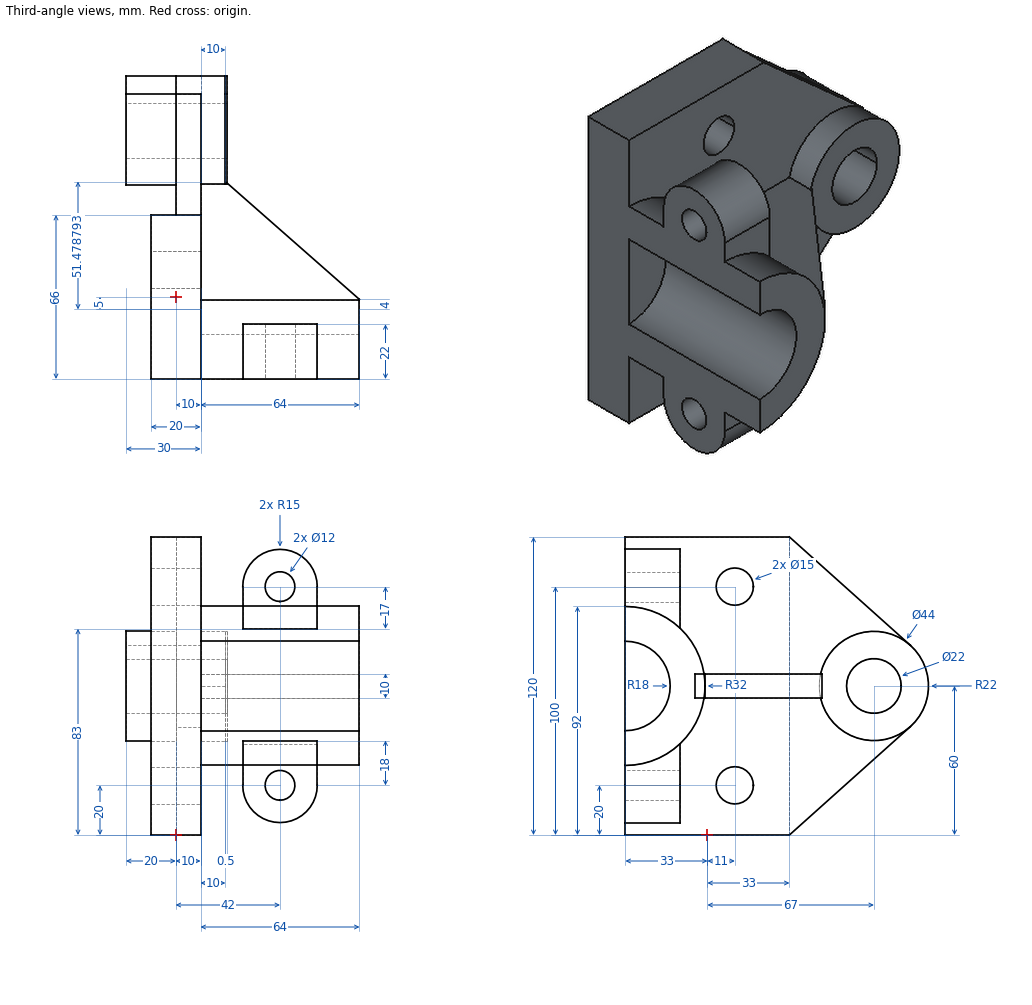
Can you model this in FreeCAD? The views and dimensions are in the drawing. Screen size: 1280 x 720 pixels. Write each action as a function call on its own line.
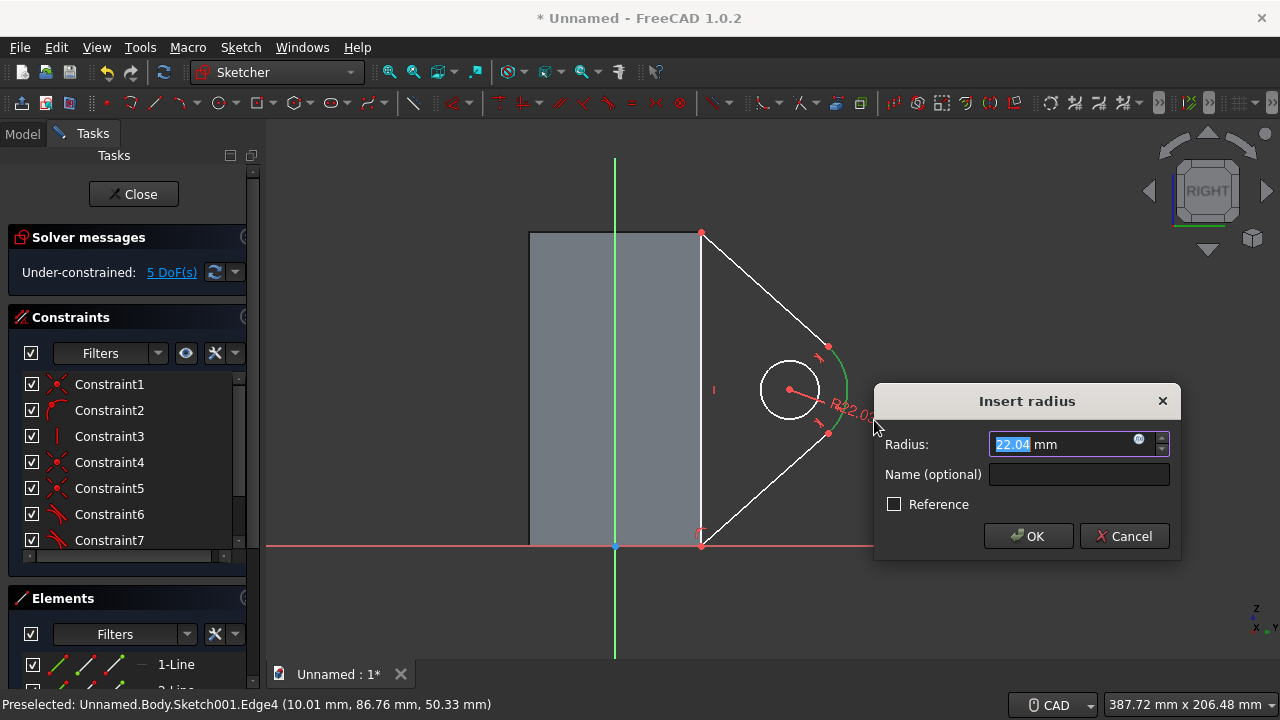
text(22)
key(Return)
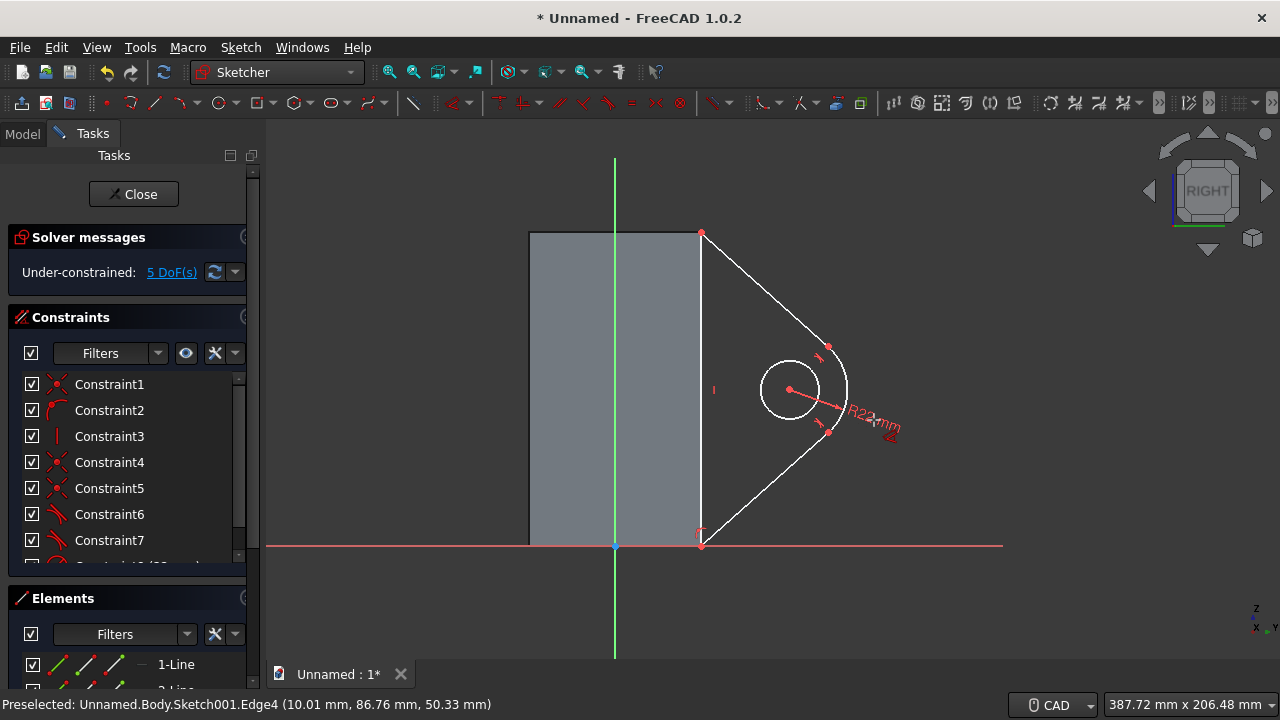
click(810, 369)
click(776, 331)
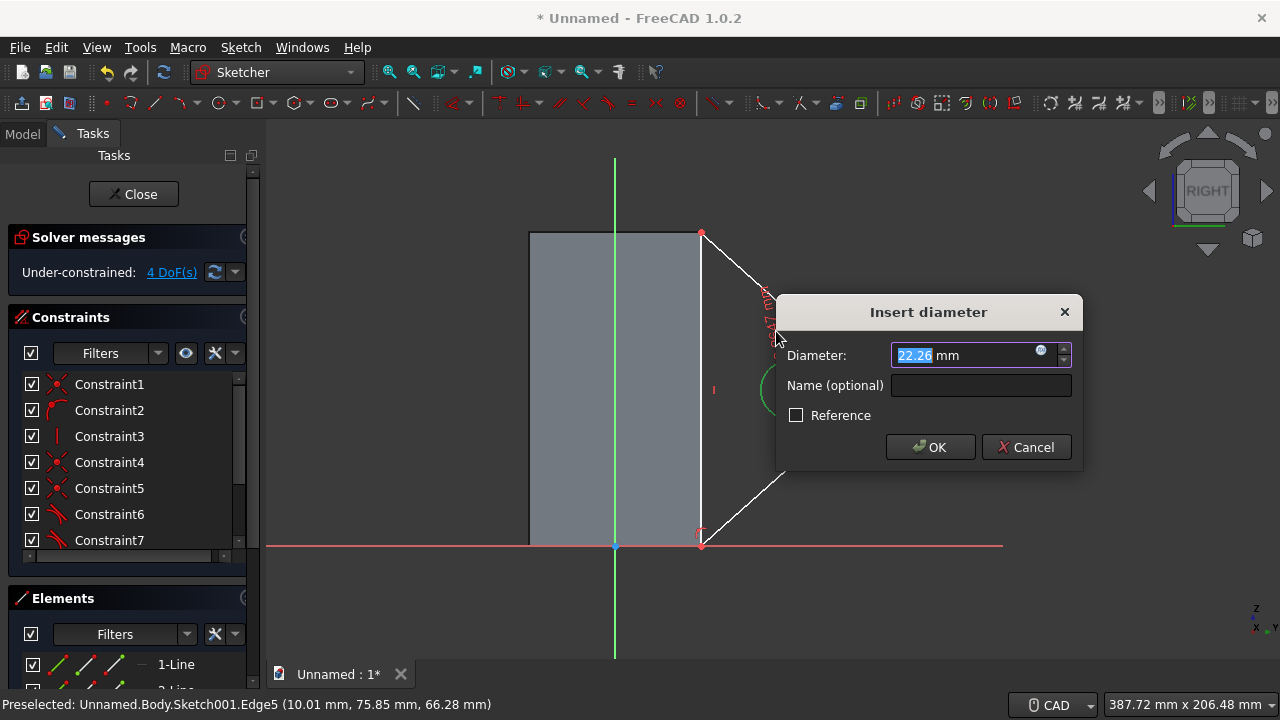
text(22)
key(Return)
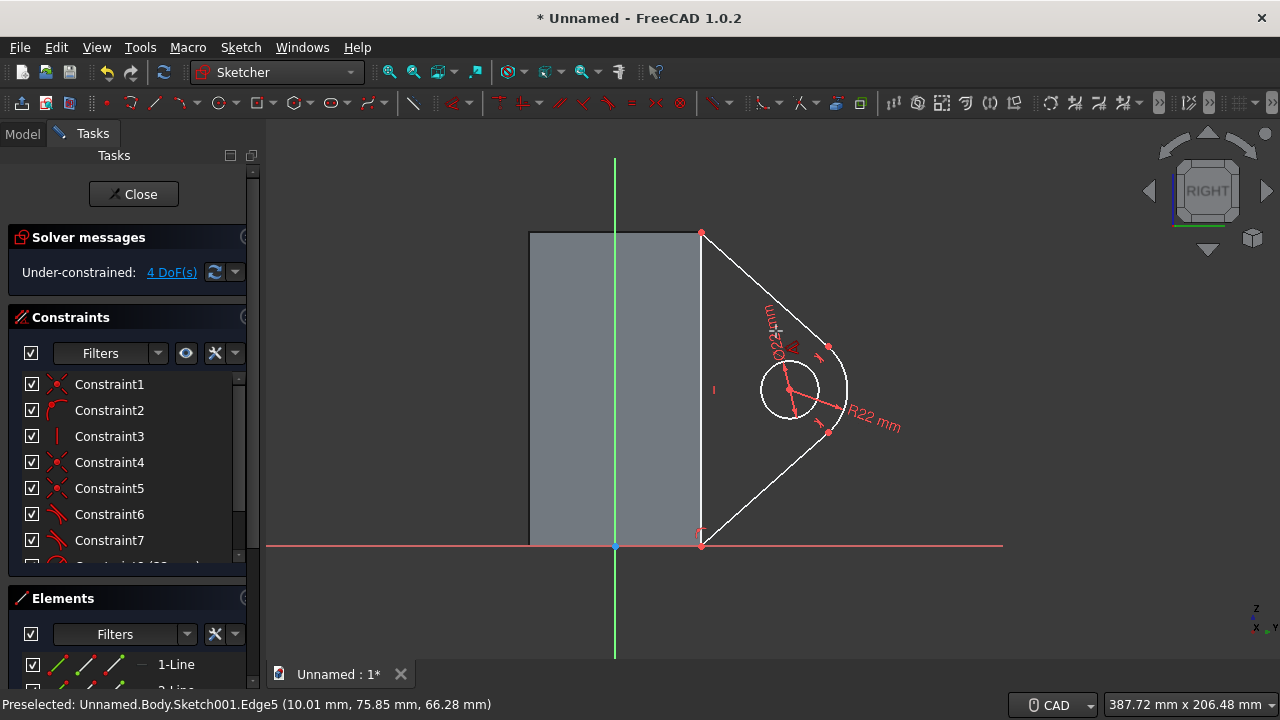
click(790, 390)
click(703, 580)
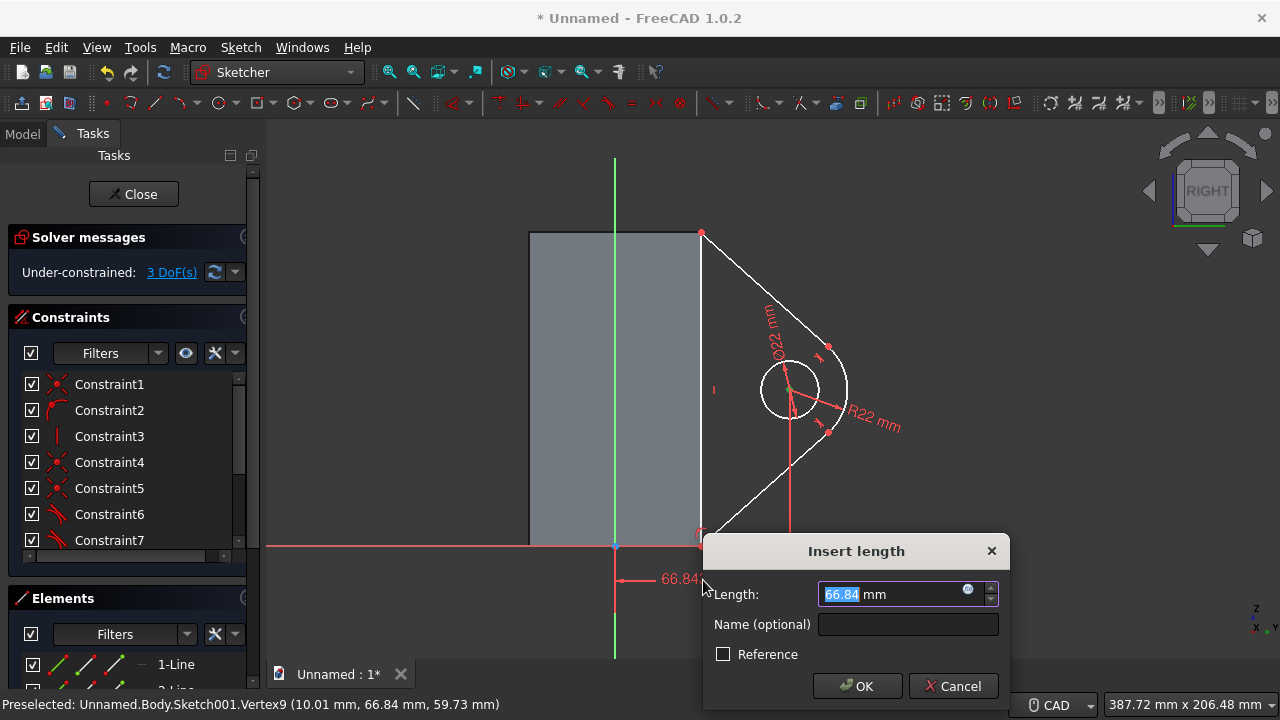
text(67)
key(Return)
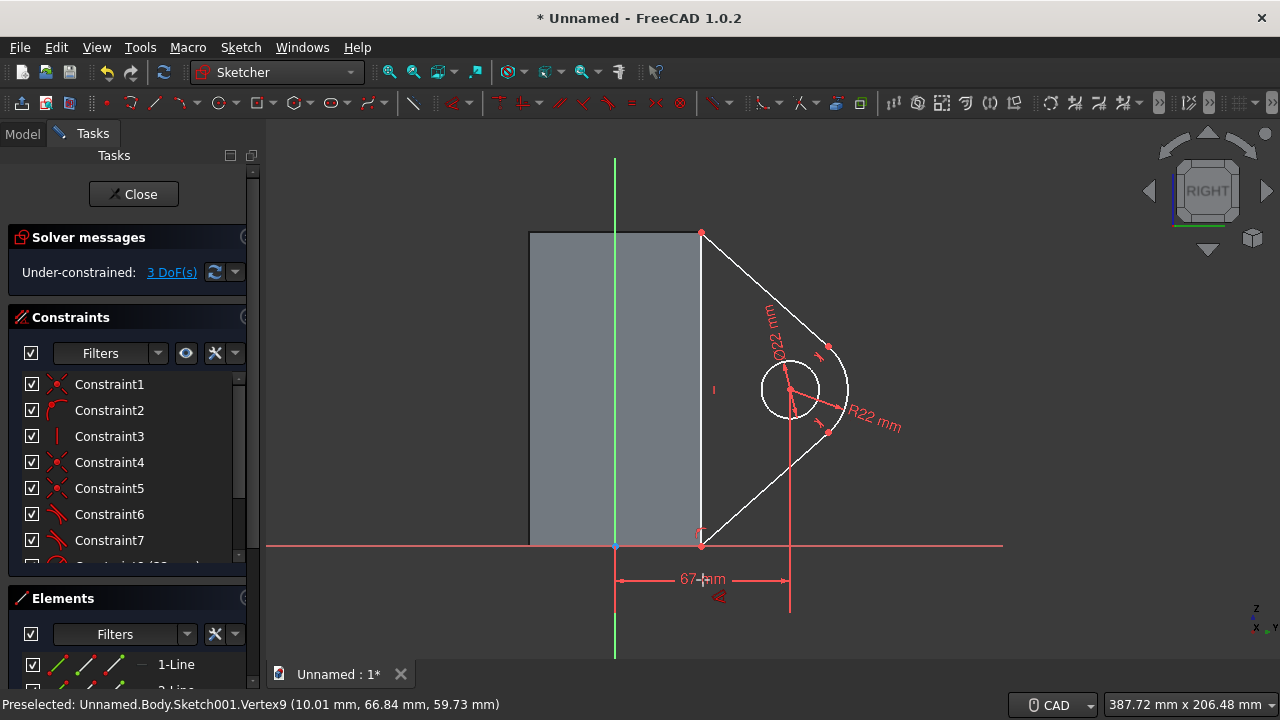
click(790, 390)
click(581, 468)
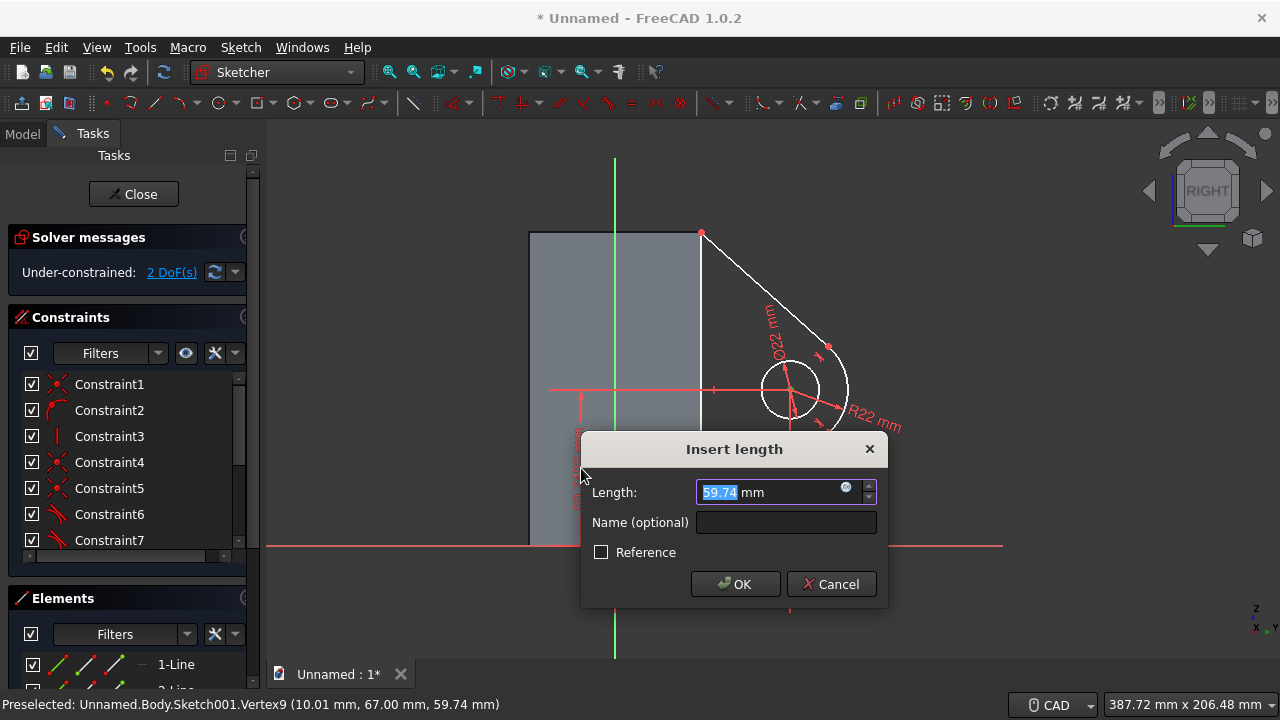
text(60)
key(Return)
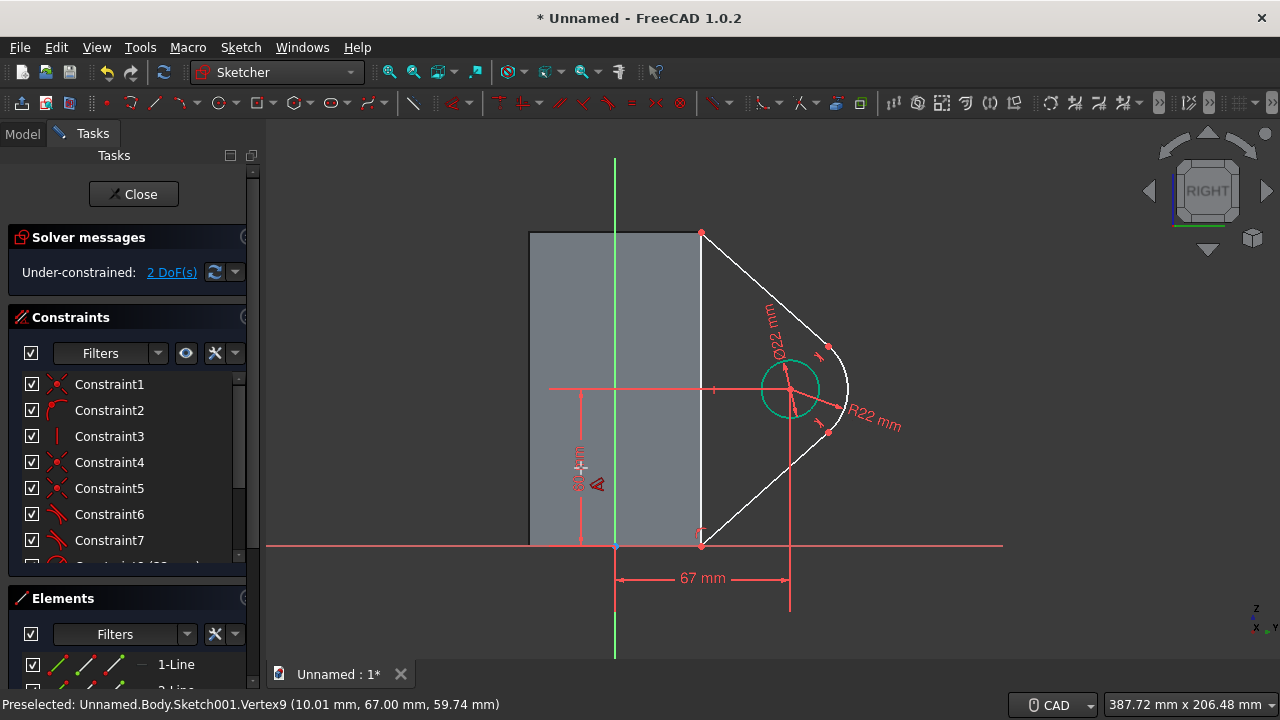
click(701, 327)
click(667, 390)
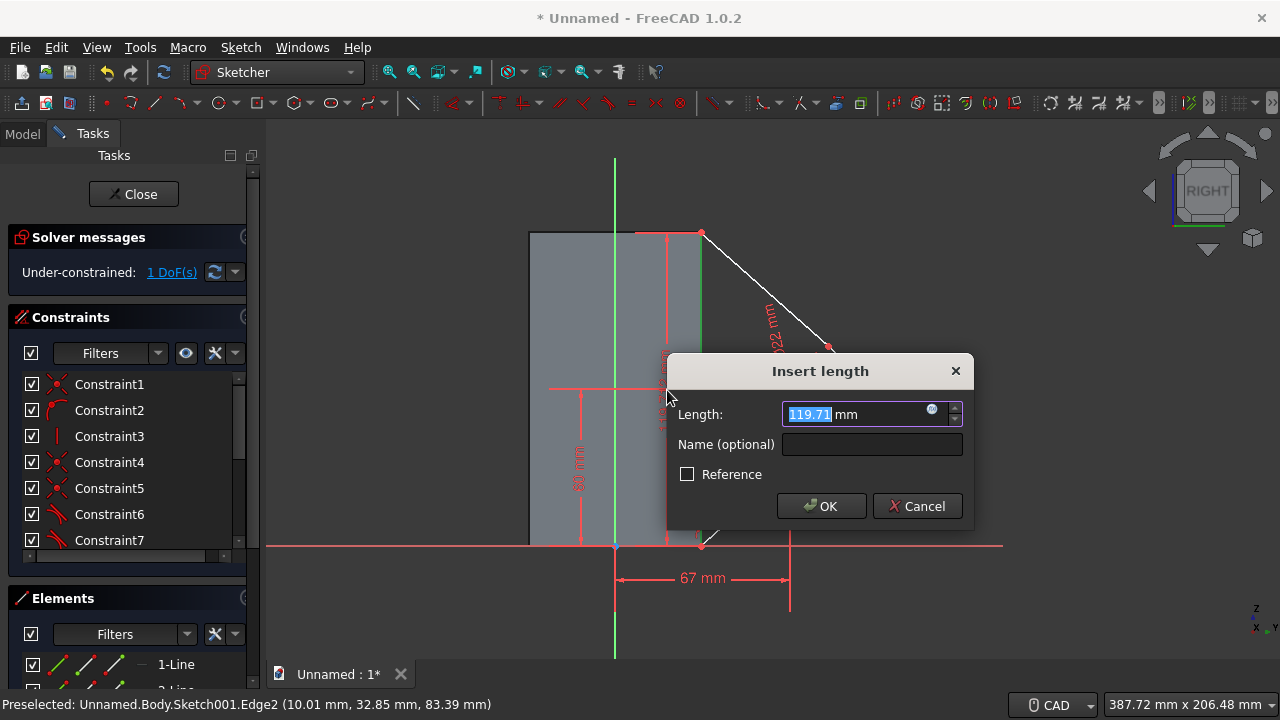
text(120)
key(Return)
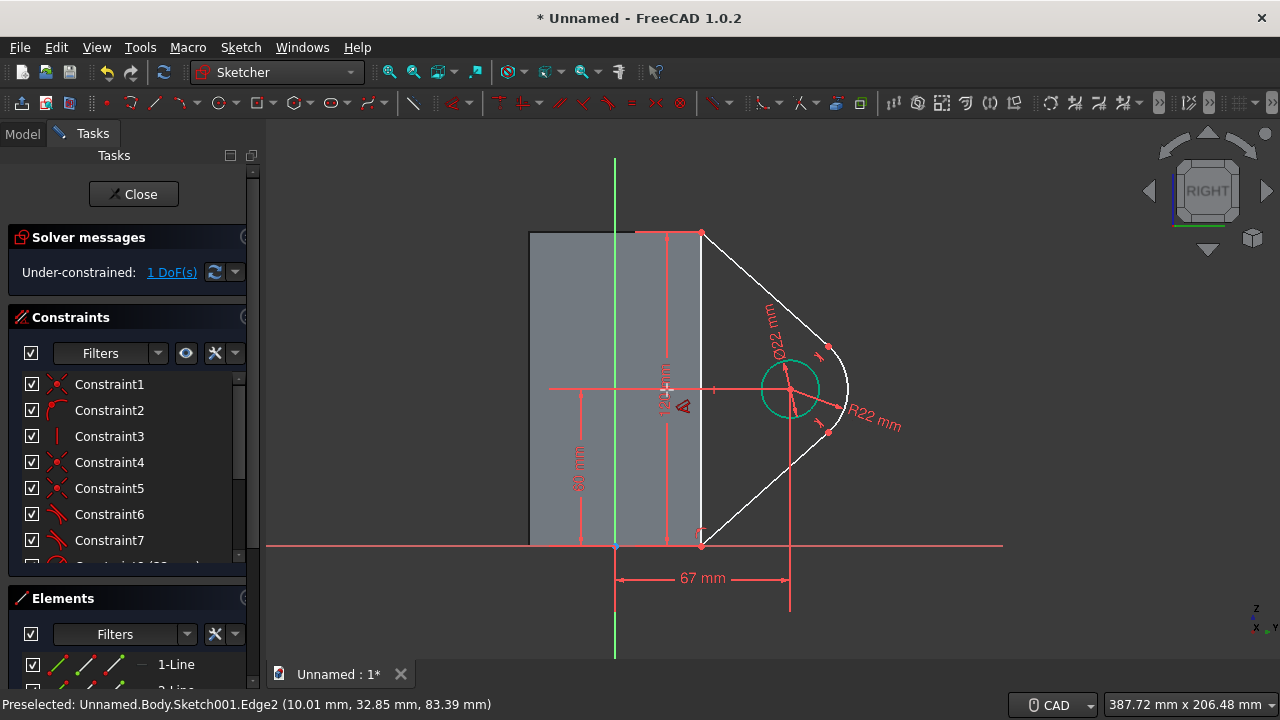
click(701, 232)
click(658, 198)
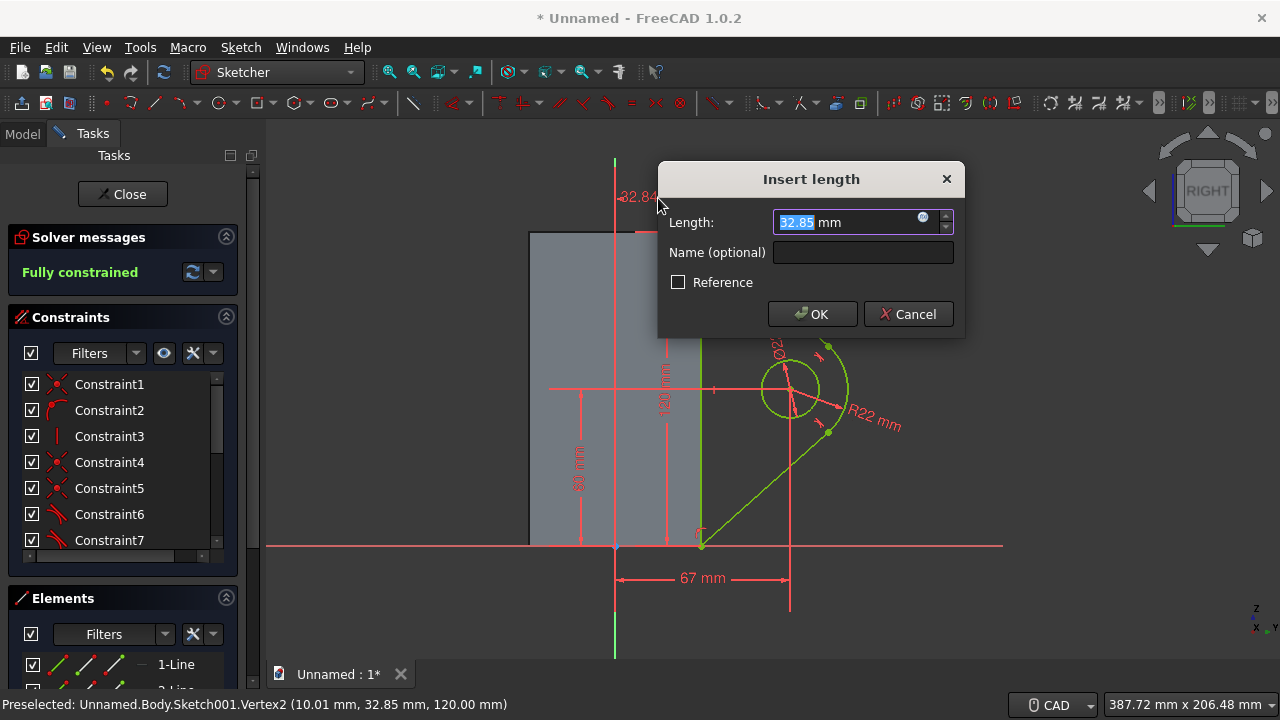
text(33)
key(Return)
key(Escape)